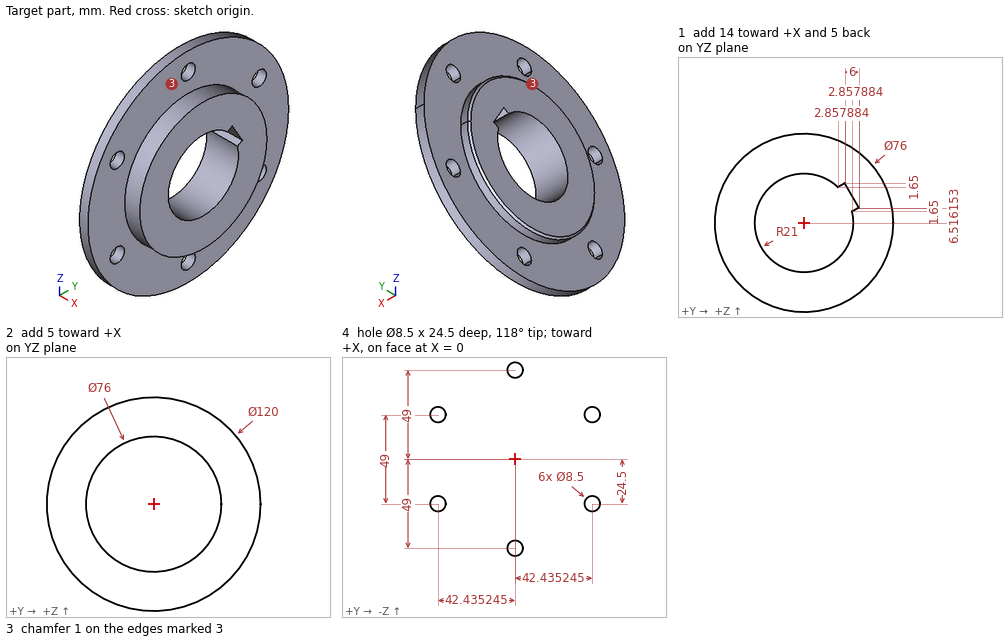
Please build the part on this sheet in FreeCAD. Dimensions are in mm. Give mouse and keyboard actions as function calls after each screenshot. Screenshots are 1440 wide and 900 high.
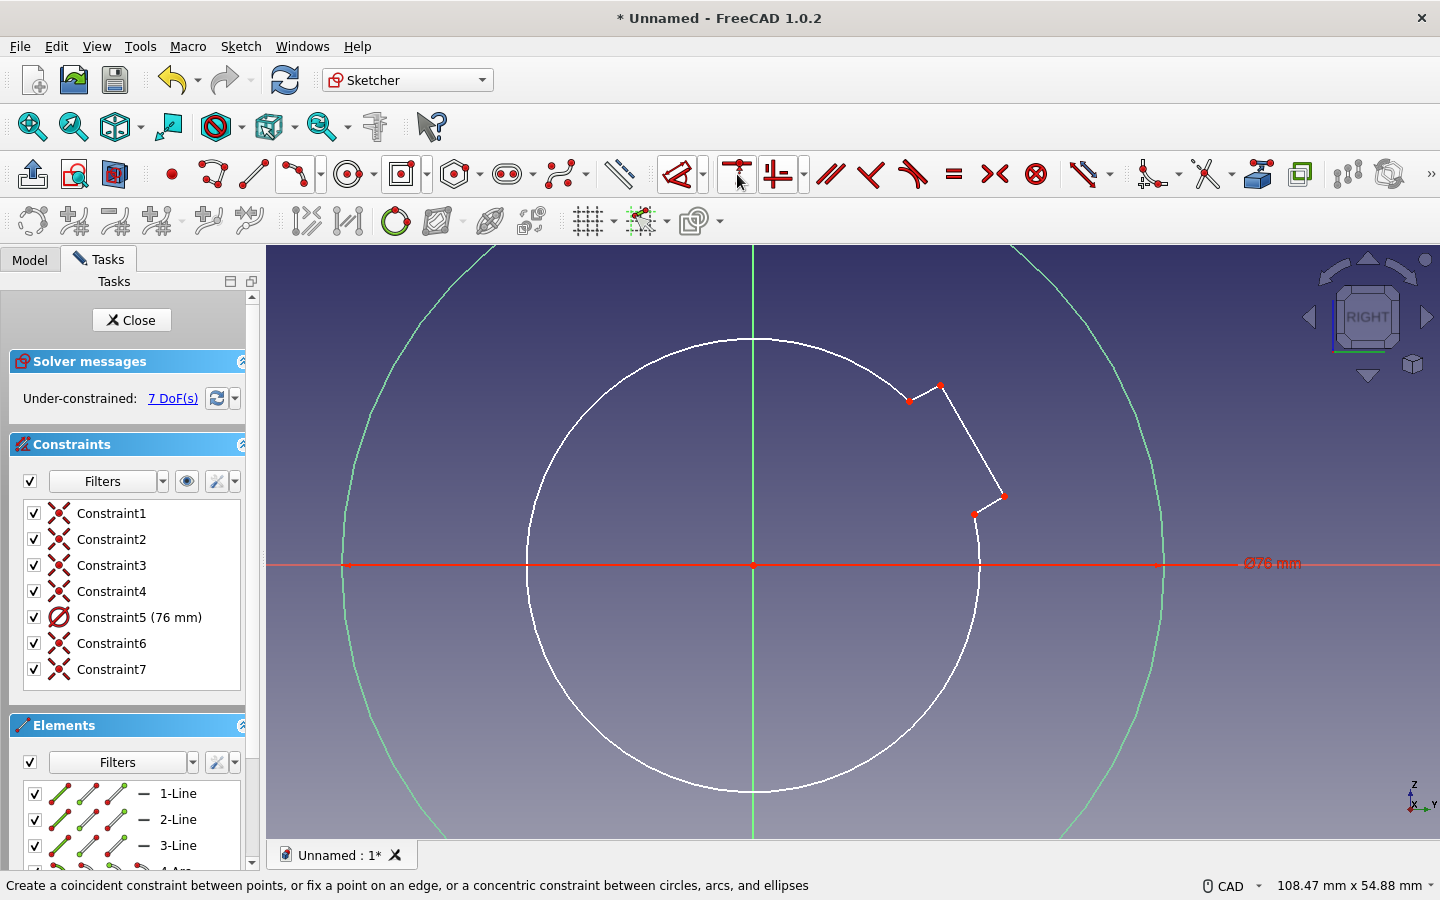
click(569, 433)
click(543, 414)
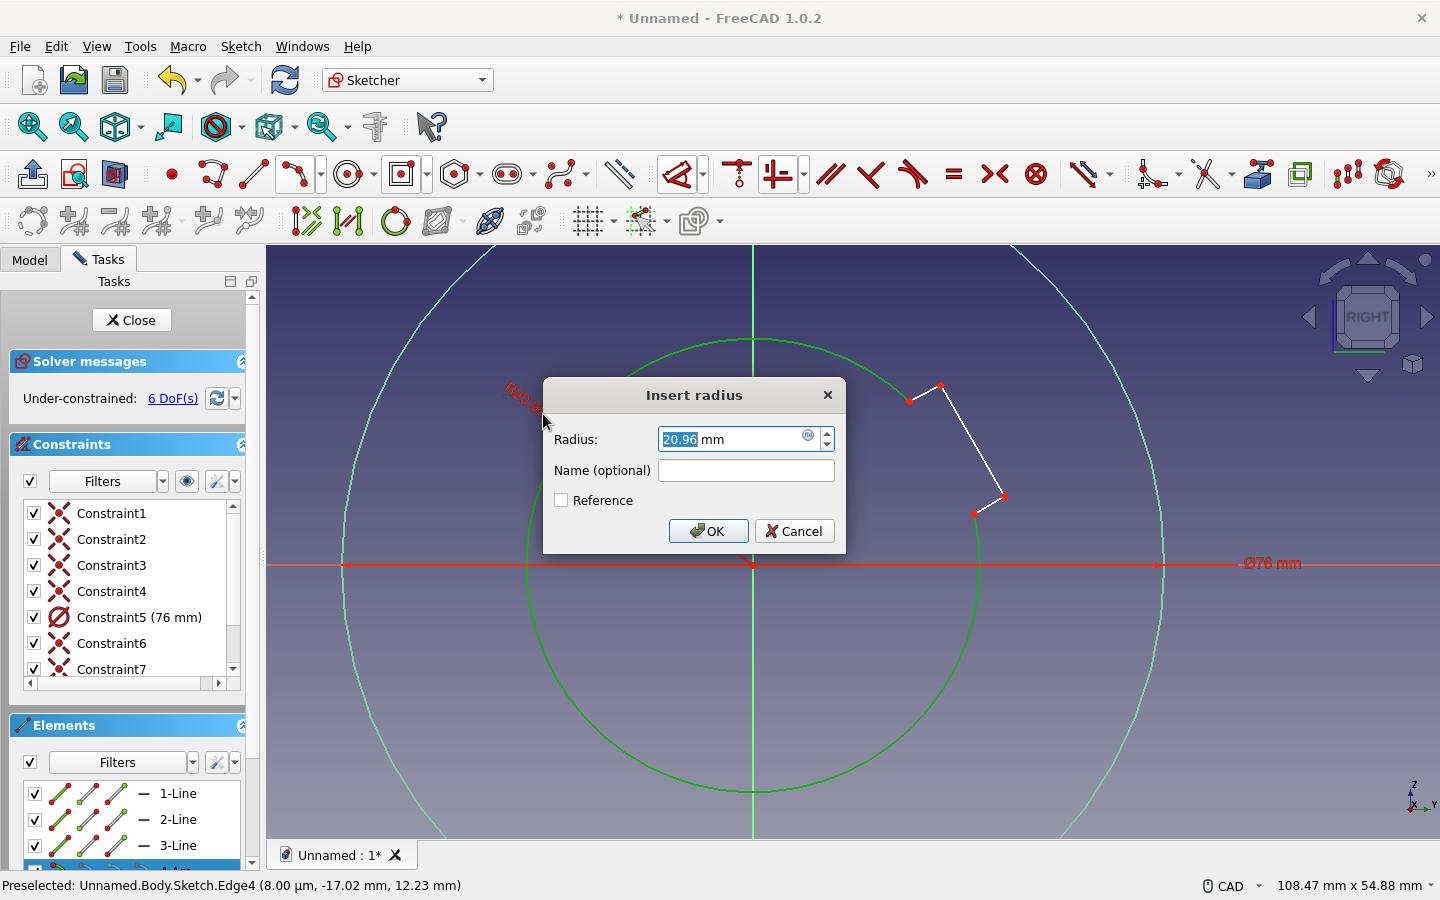
text(21)
key(Return)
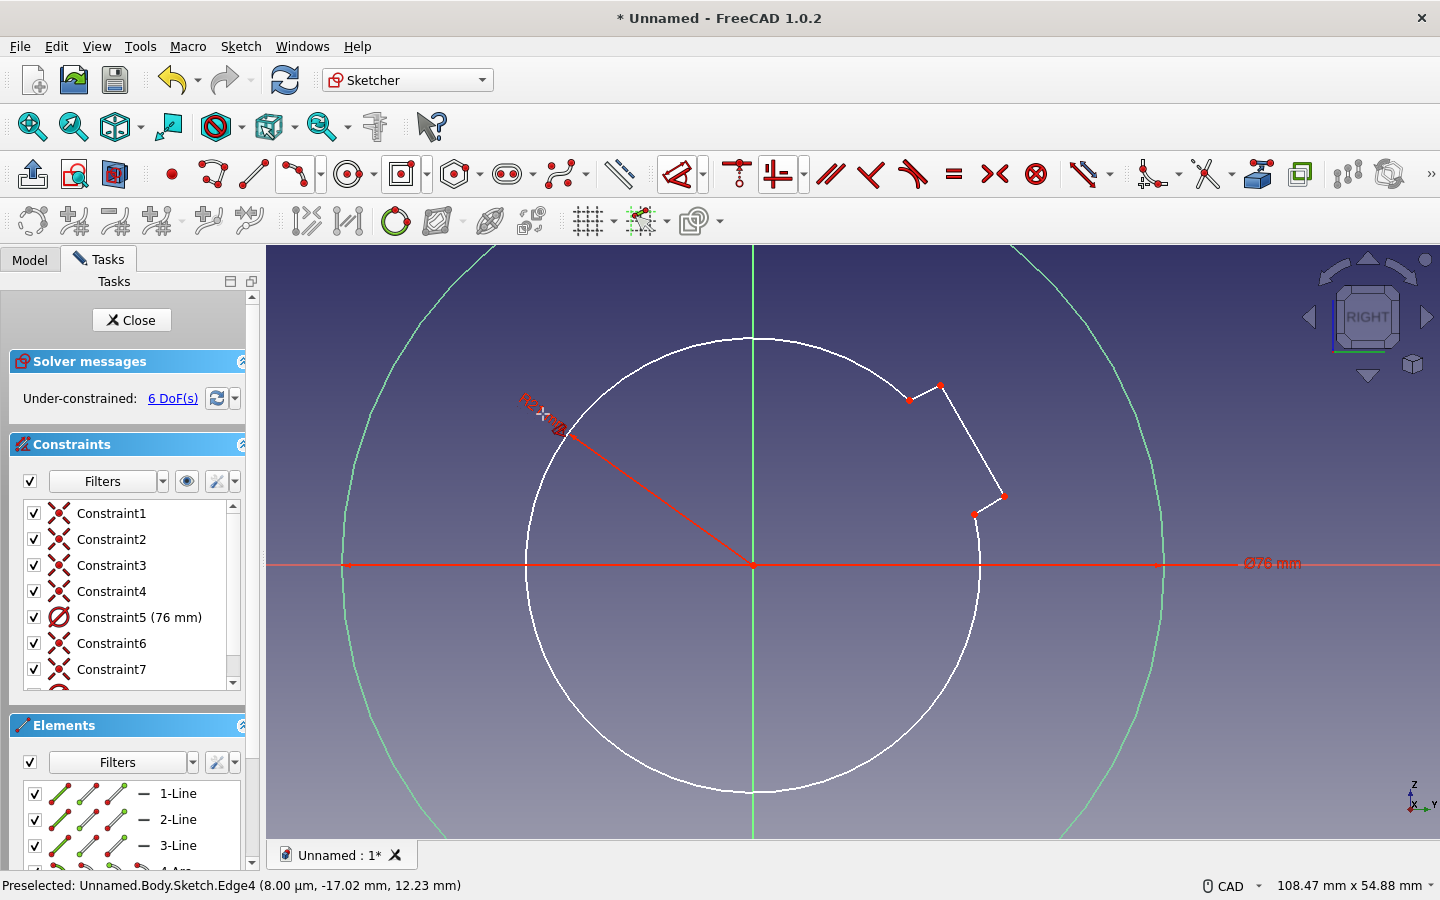
click(960, 418)
click(973, 351)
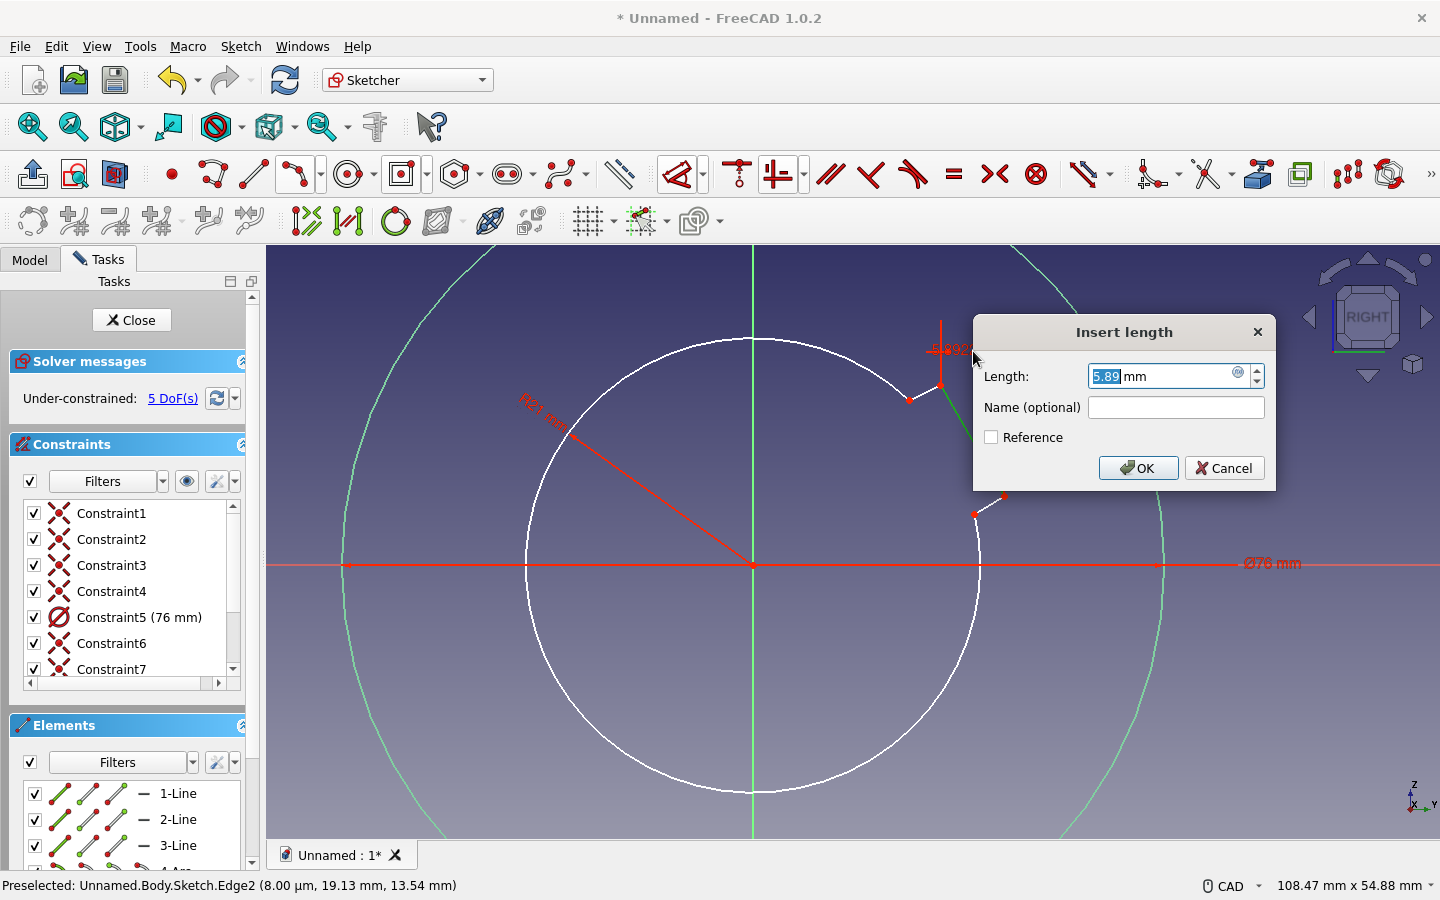
text(6)
key(Return)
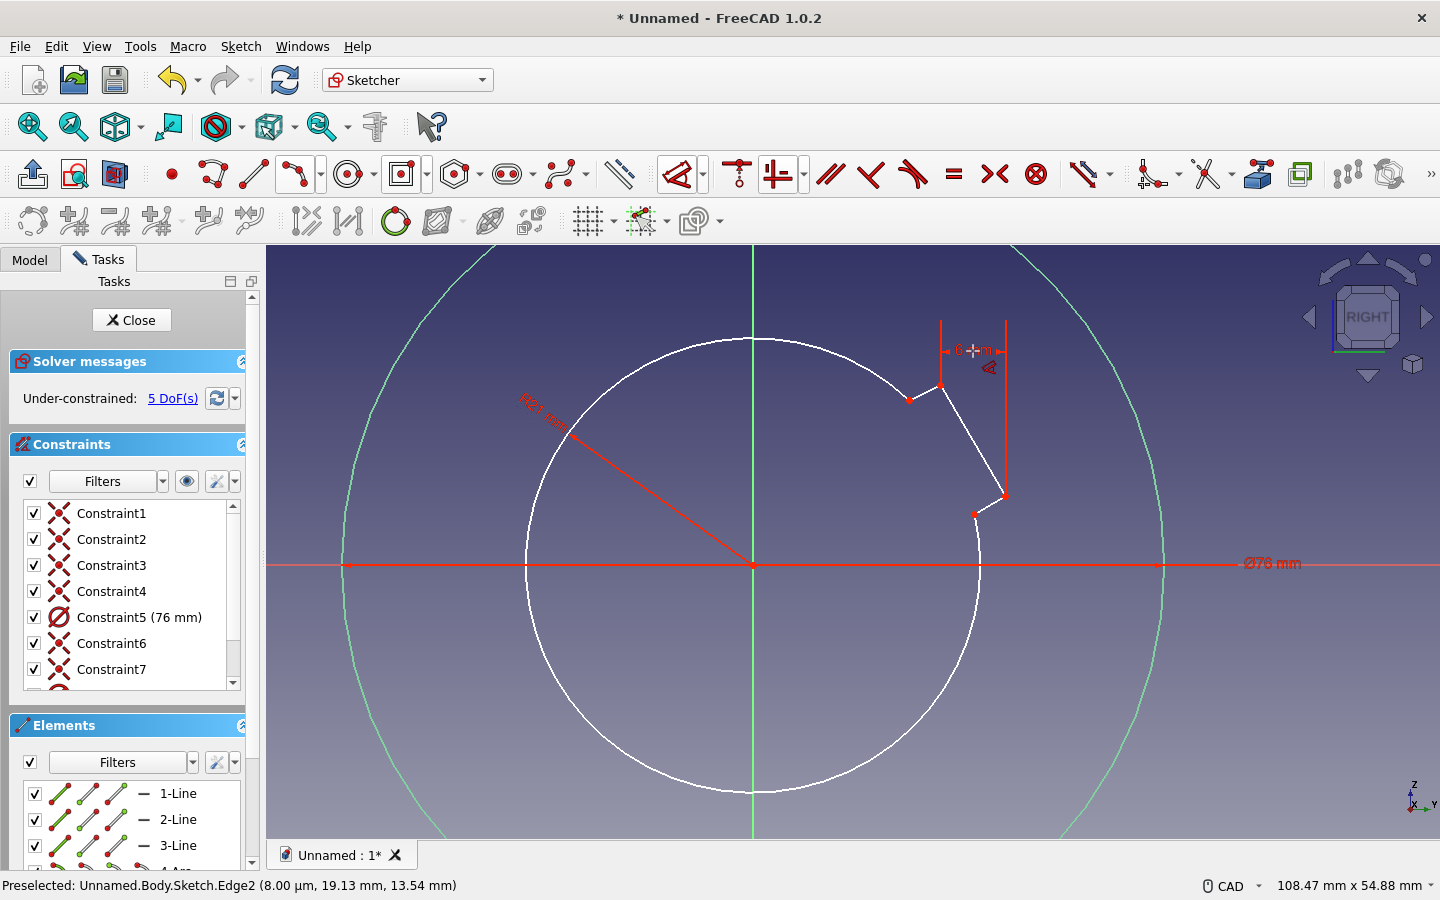
scroll(919, 396, up, 4)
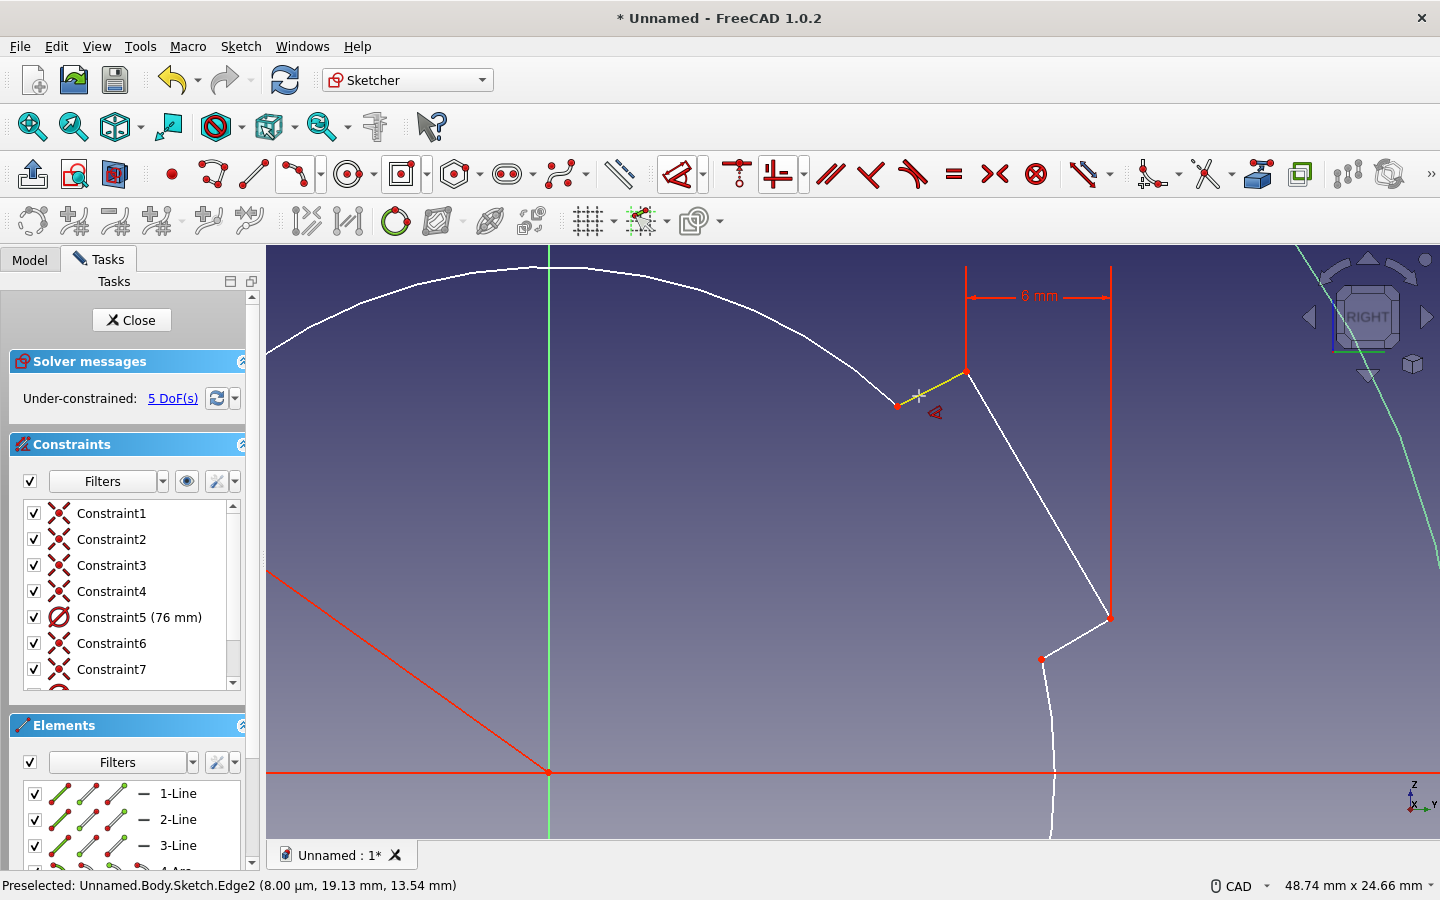
click(918, 396)
click(1000, 389)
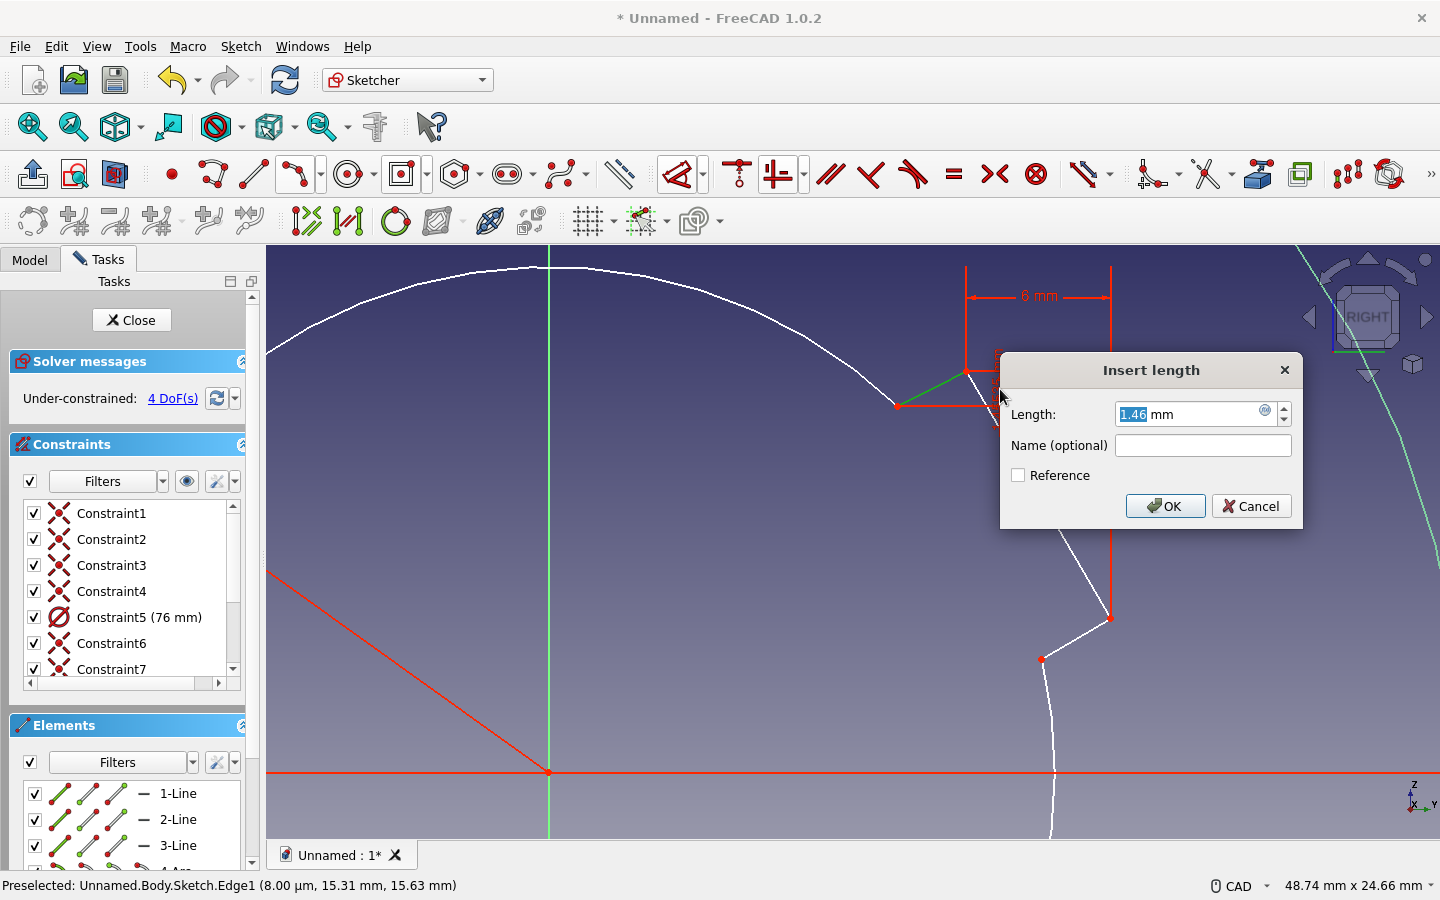
text(1.65)
key(Return)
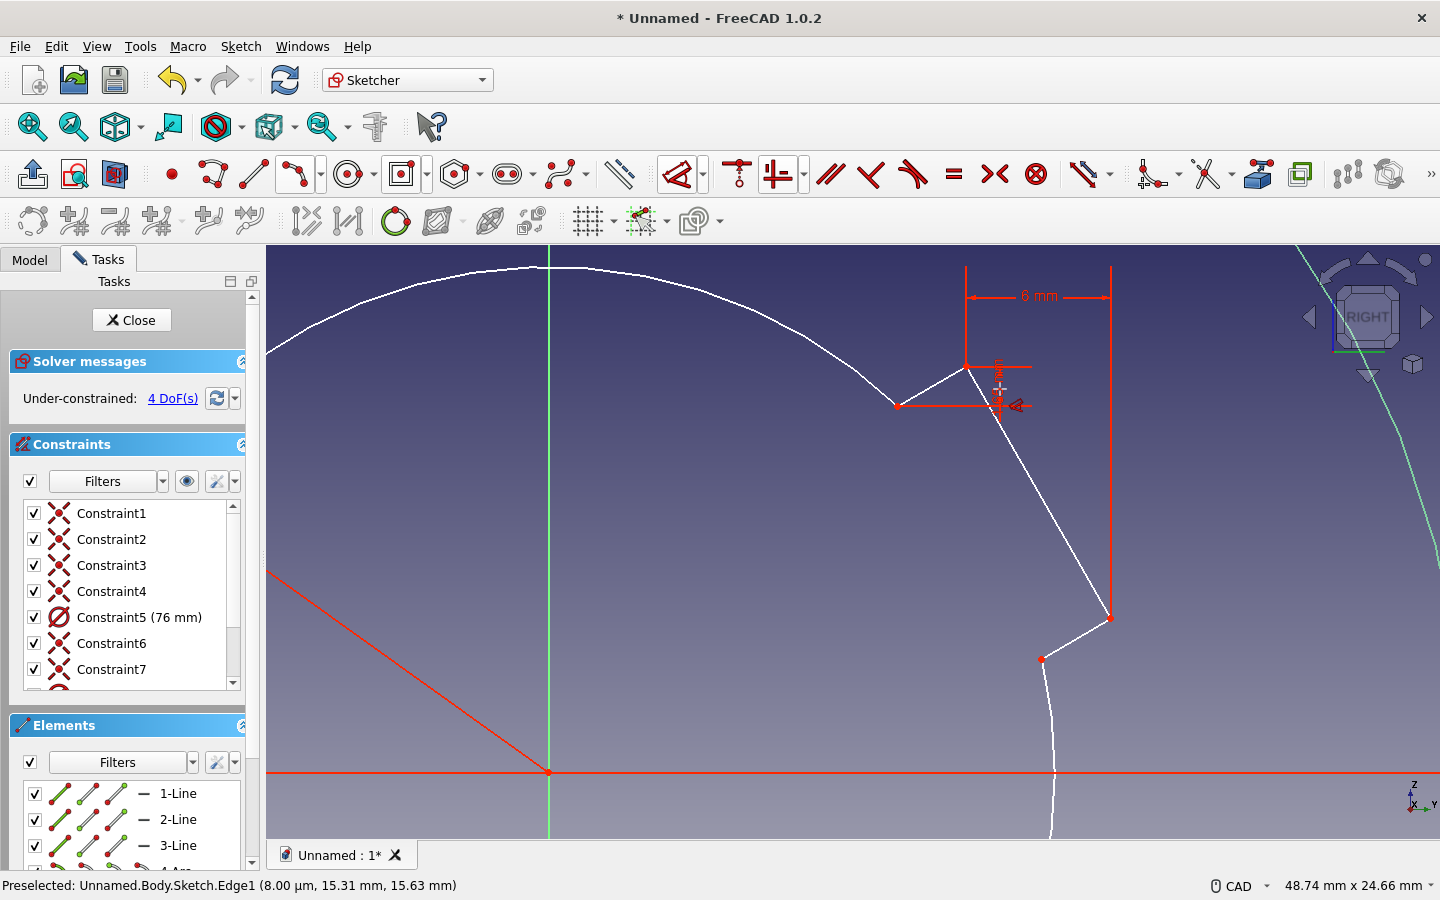
click(1090, 631)
click(1145, 639)